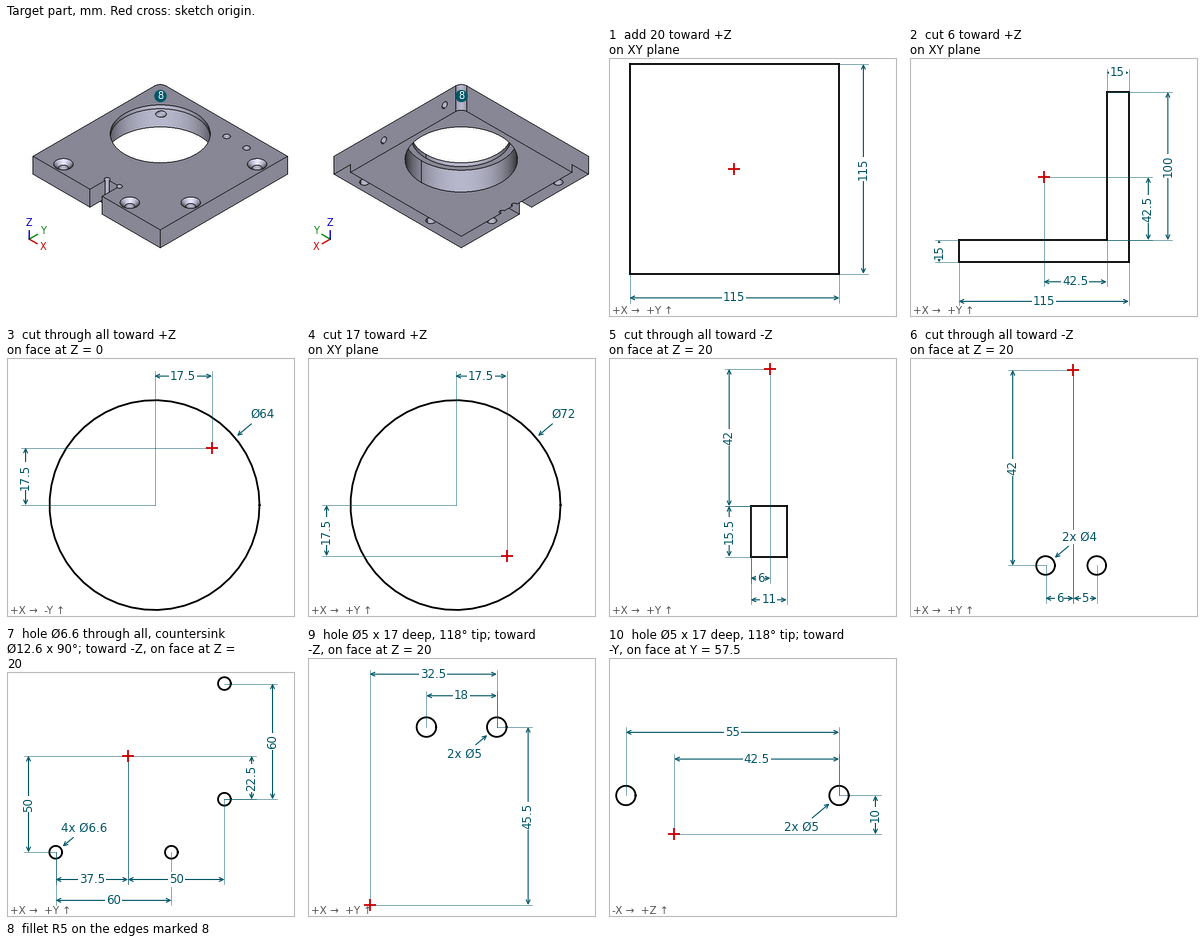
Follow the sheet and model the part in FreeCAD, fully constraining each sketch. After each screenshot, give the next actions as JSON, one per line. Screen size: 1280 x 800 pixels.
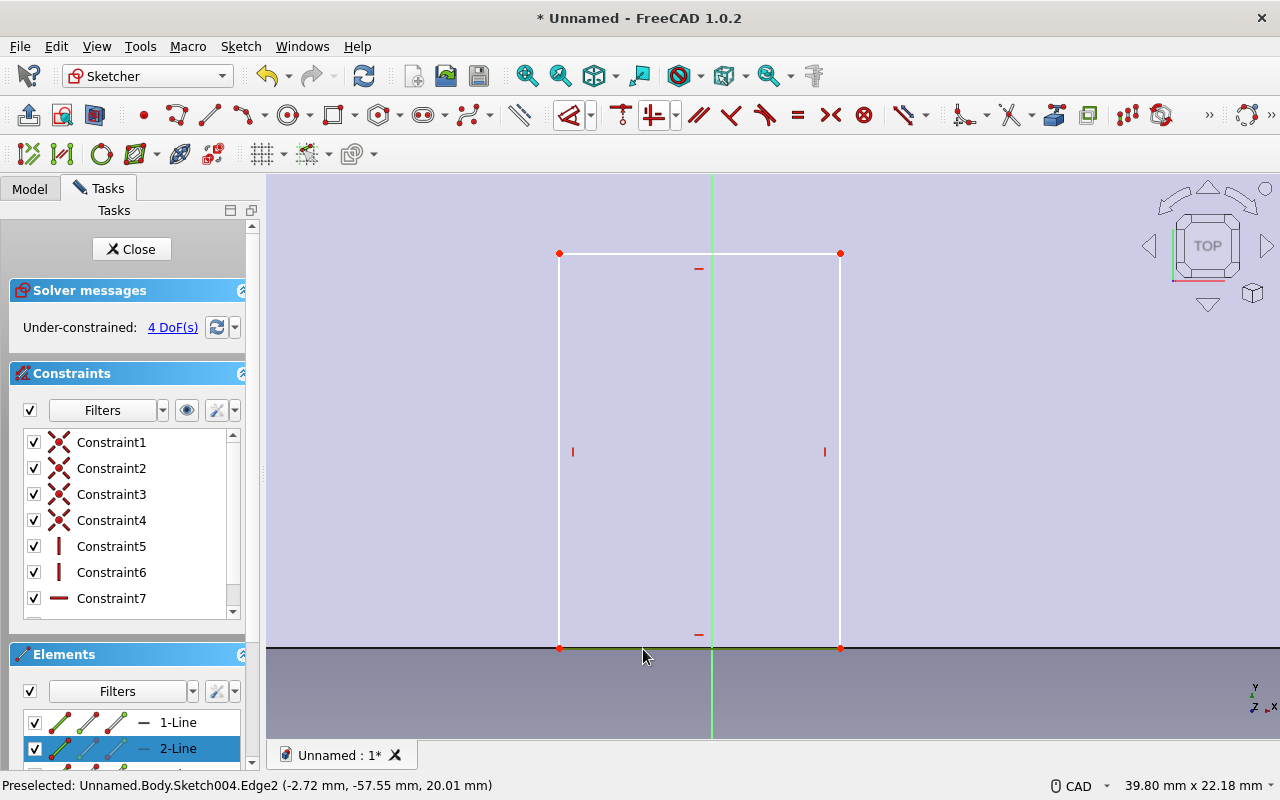
{"action": "key", "text": "l"}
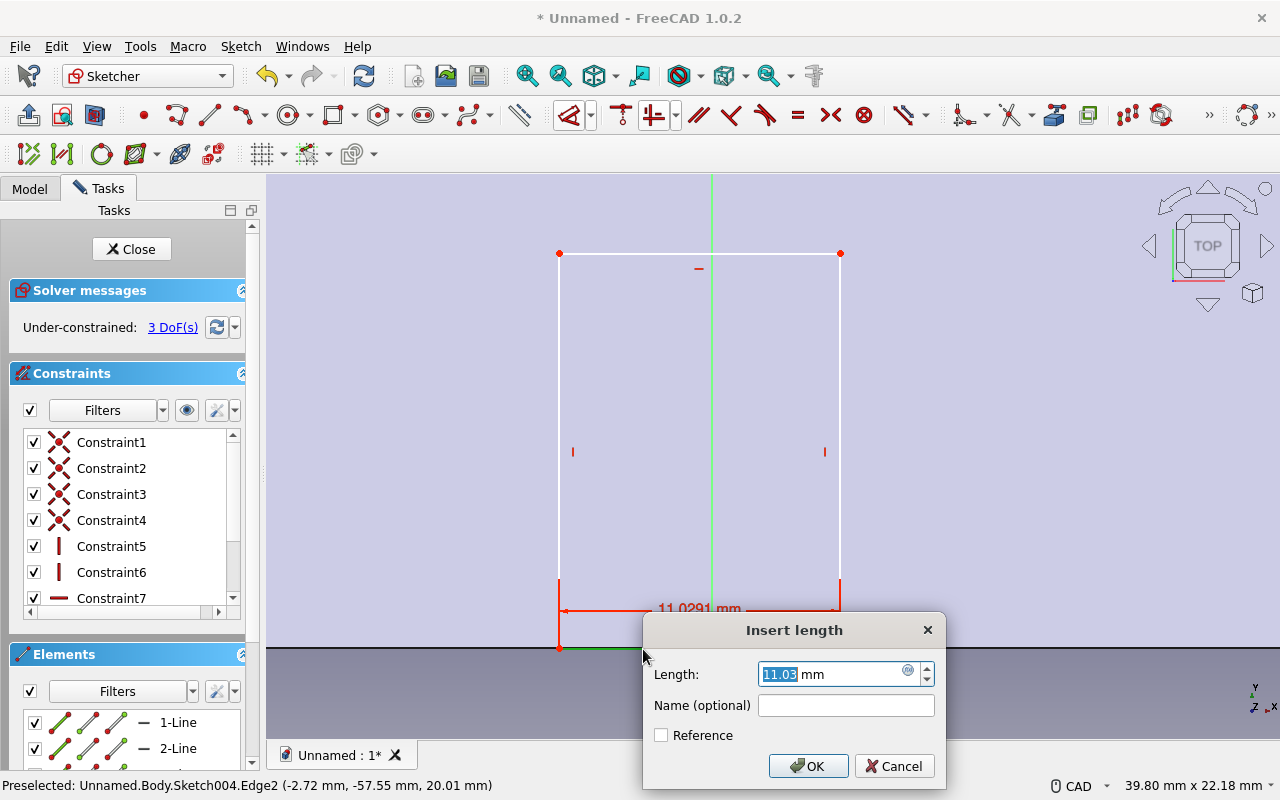
{"action": "type", "text": "11"}
{"action": "key", "text": "Return"}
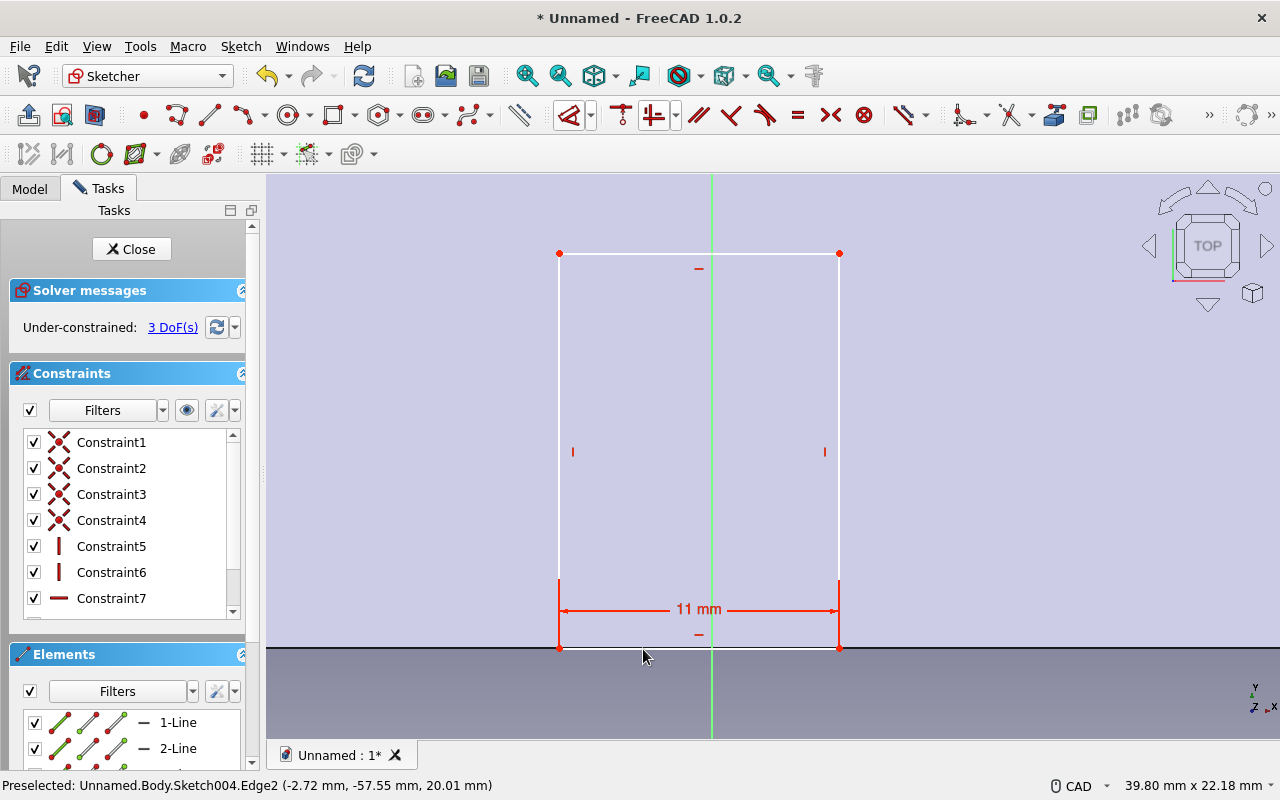
{"action": "left_click", "coordinate": [559, 254]}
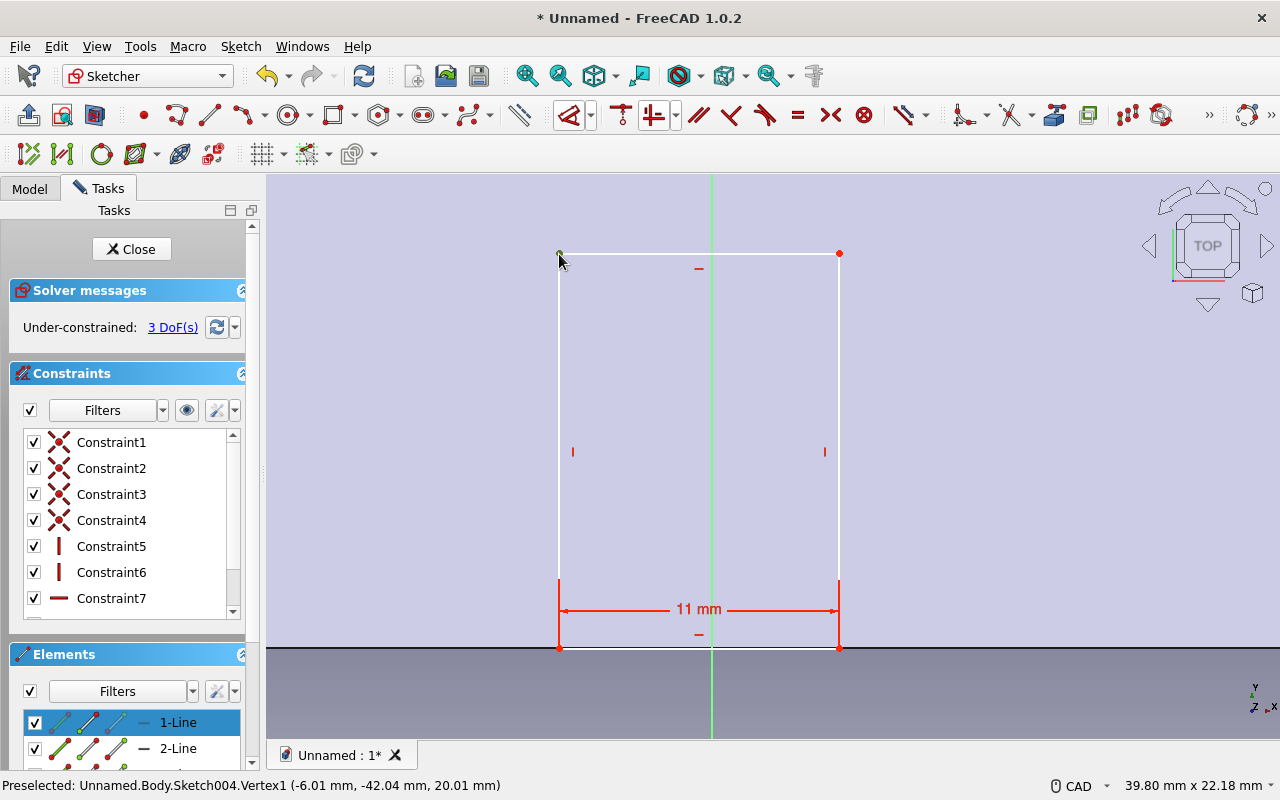
{"action": "key", "text": "l"}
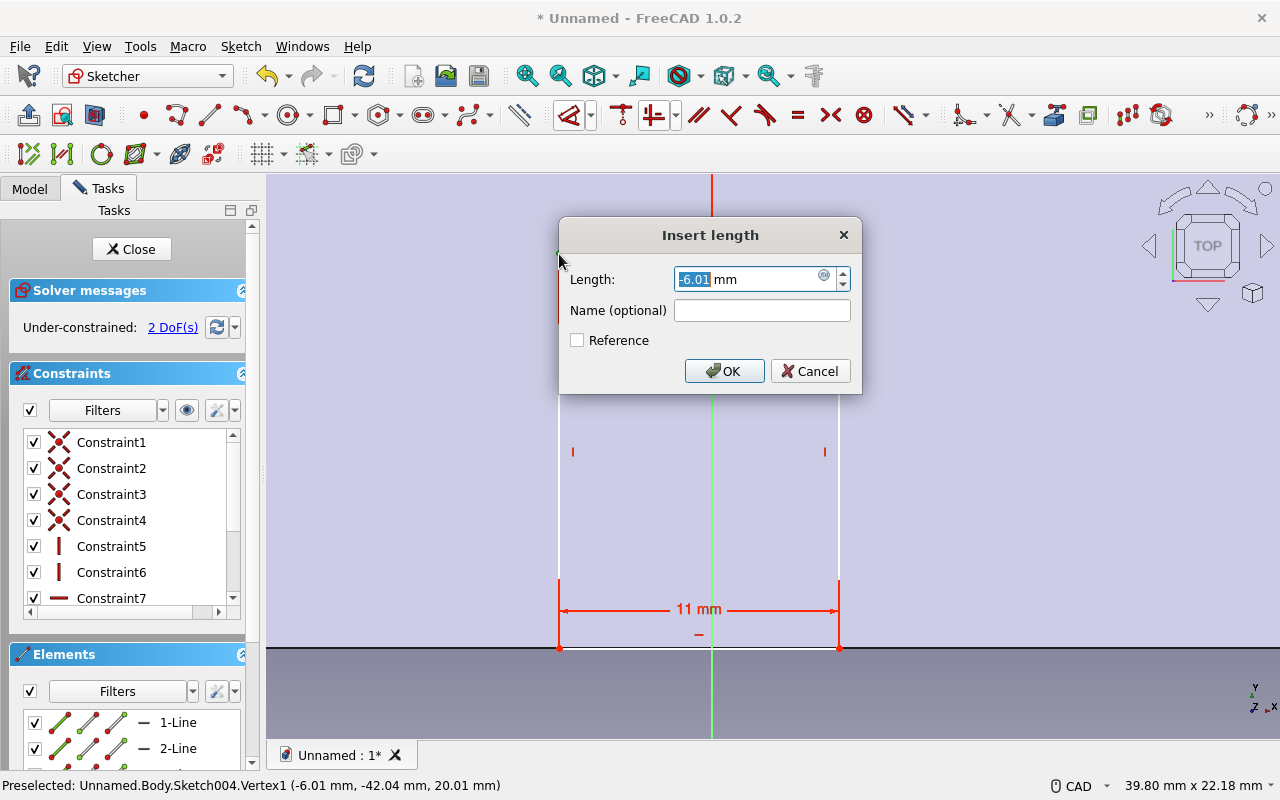
{"action": "type", "text": "-6"}
{"action": "key", "text": "Return"}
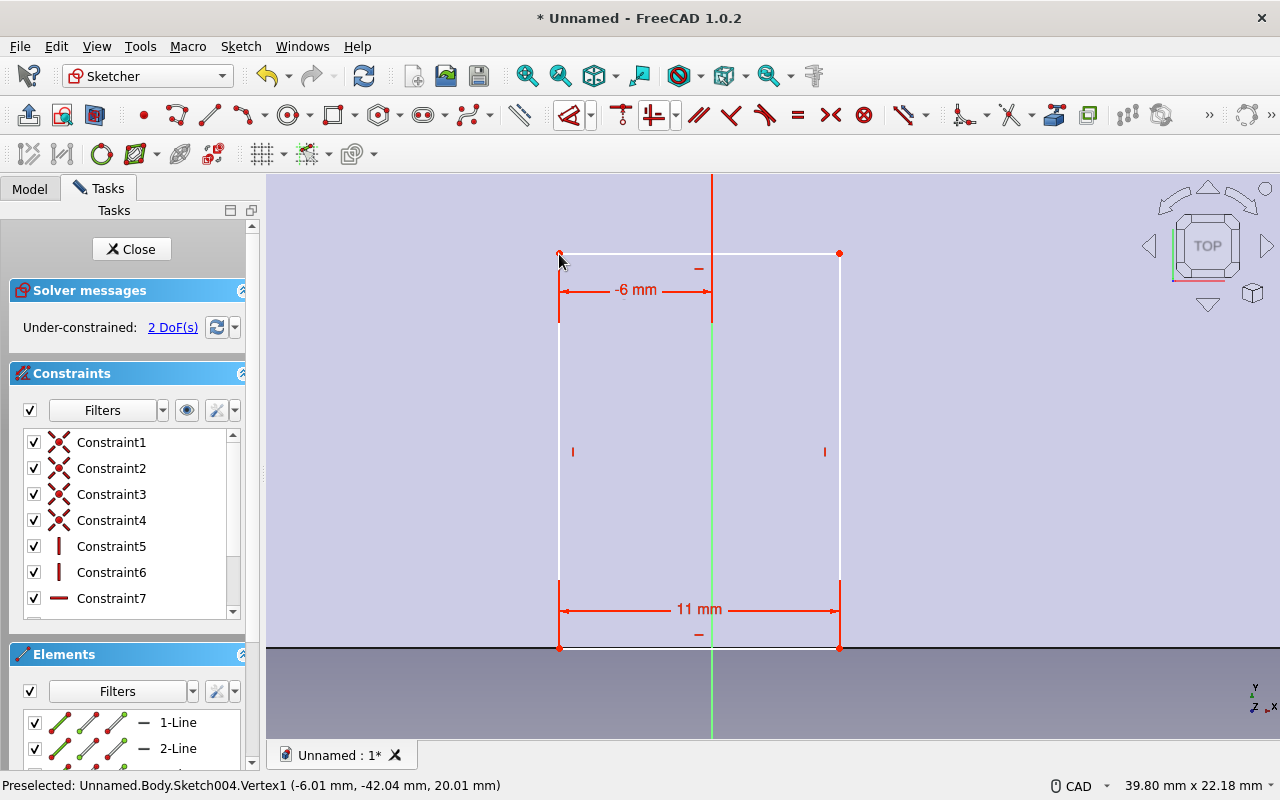
{"action": "left_click", "coordinate": [559, 254]}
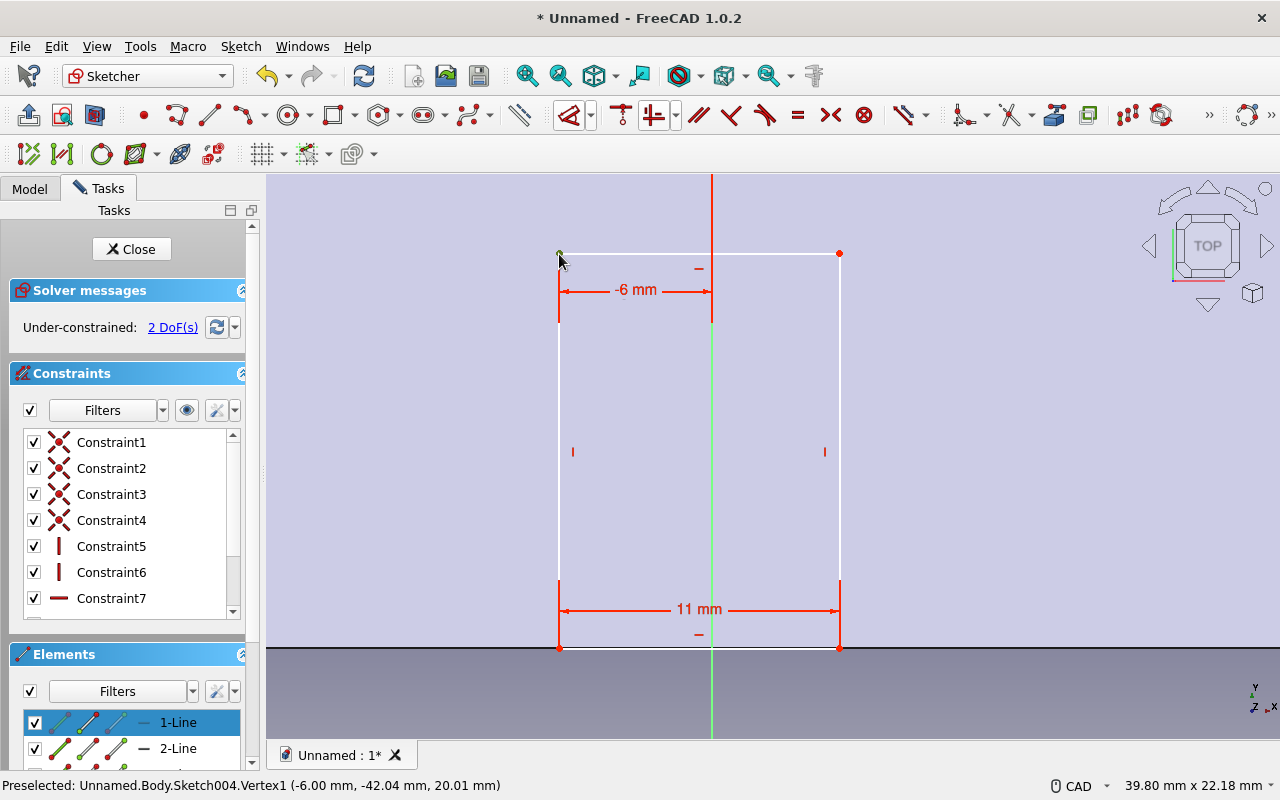
{"action": "key", "text": "i"}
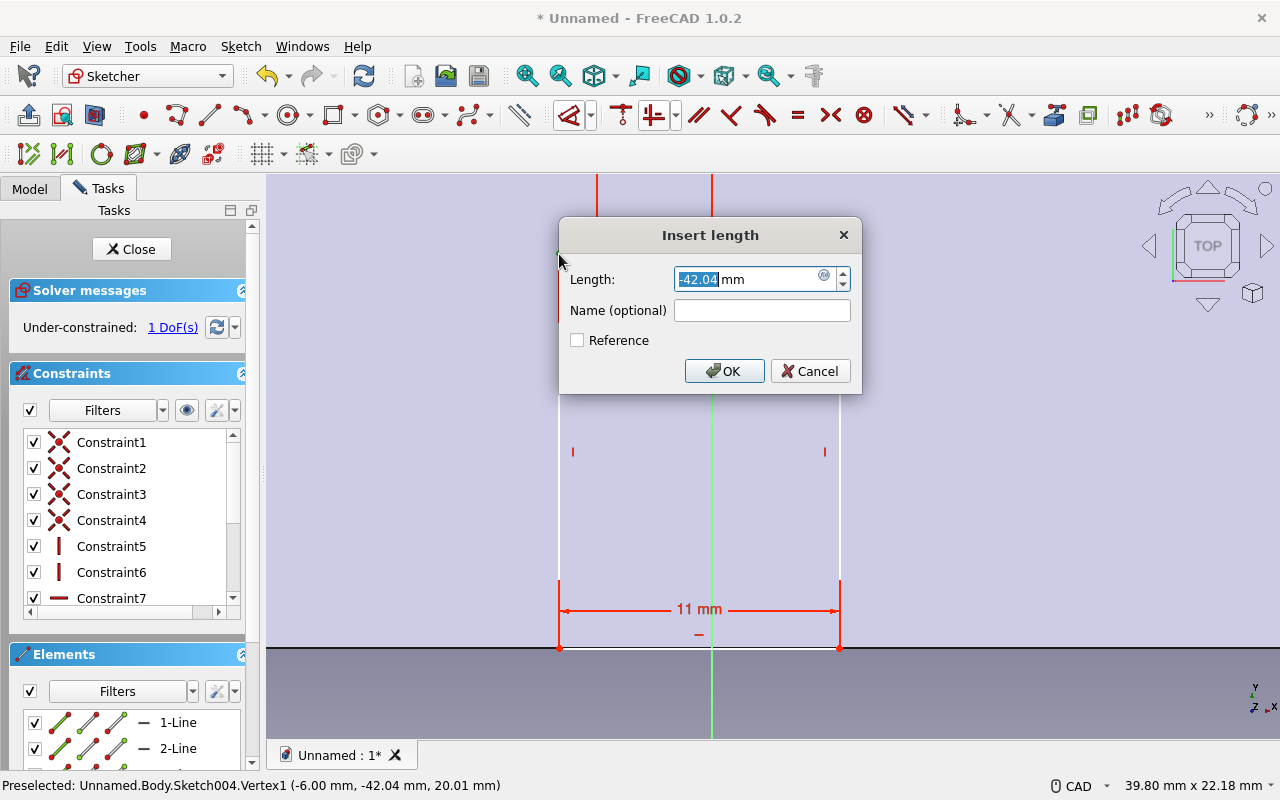
{"action": "type", "text": "-42"}
{"action": "key", "text": "Return"}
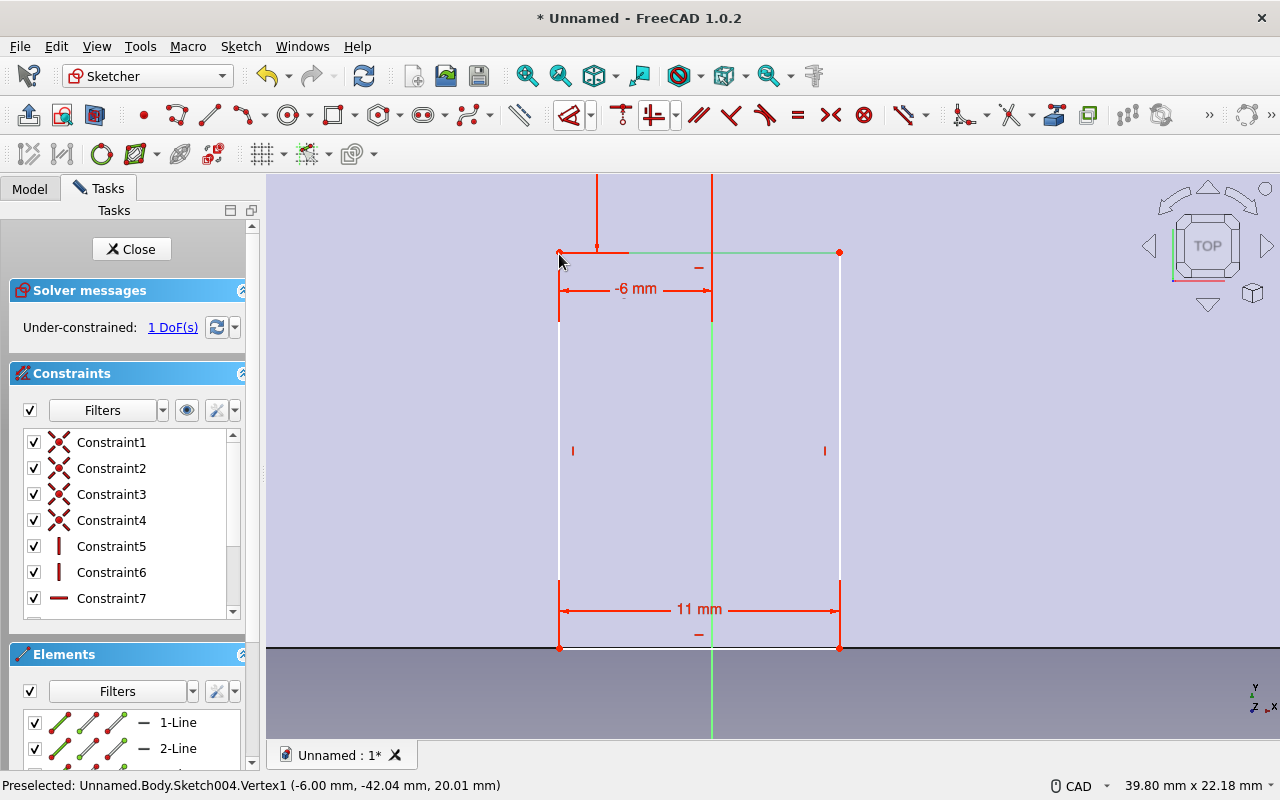
{"action": "left_click", "coordinate": [559, 372]}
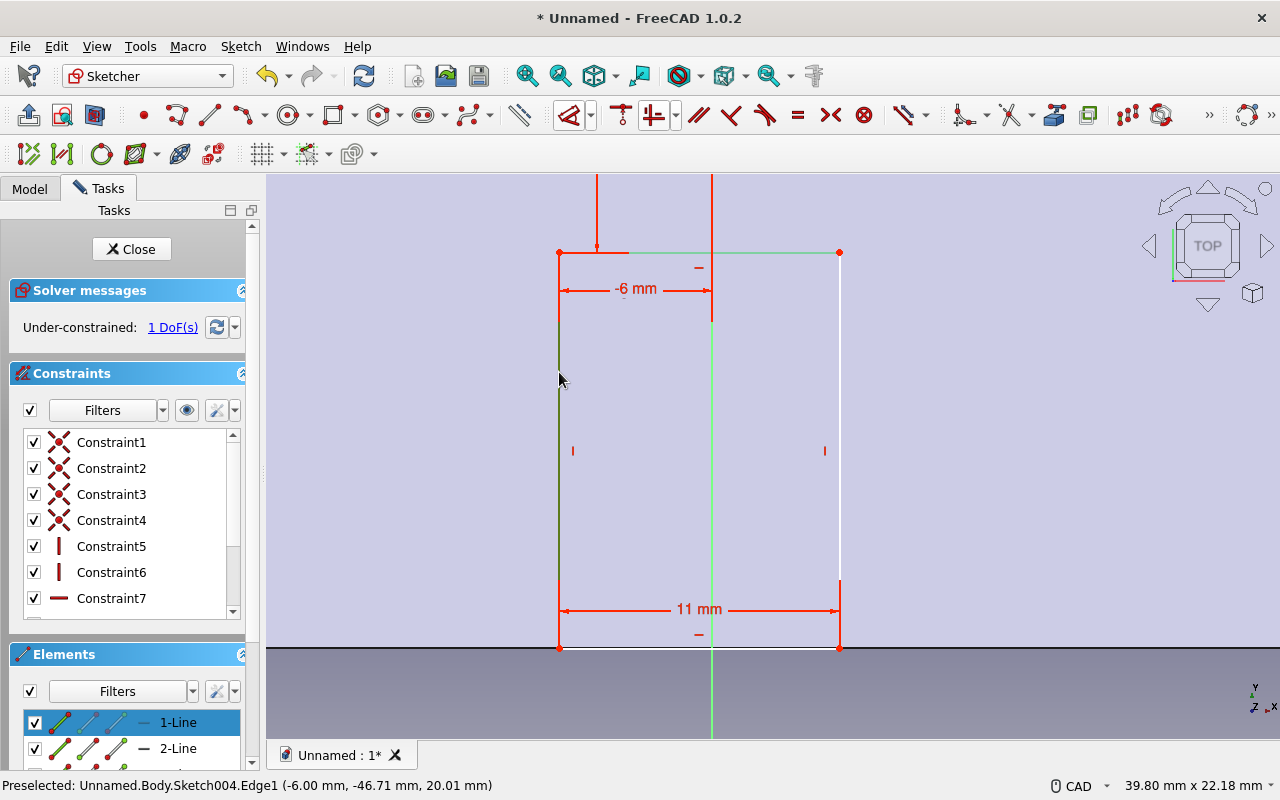
{"action": "key", "text": "i"}